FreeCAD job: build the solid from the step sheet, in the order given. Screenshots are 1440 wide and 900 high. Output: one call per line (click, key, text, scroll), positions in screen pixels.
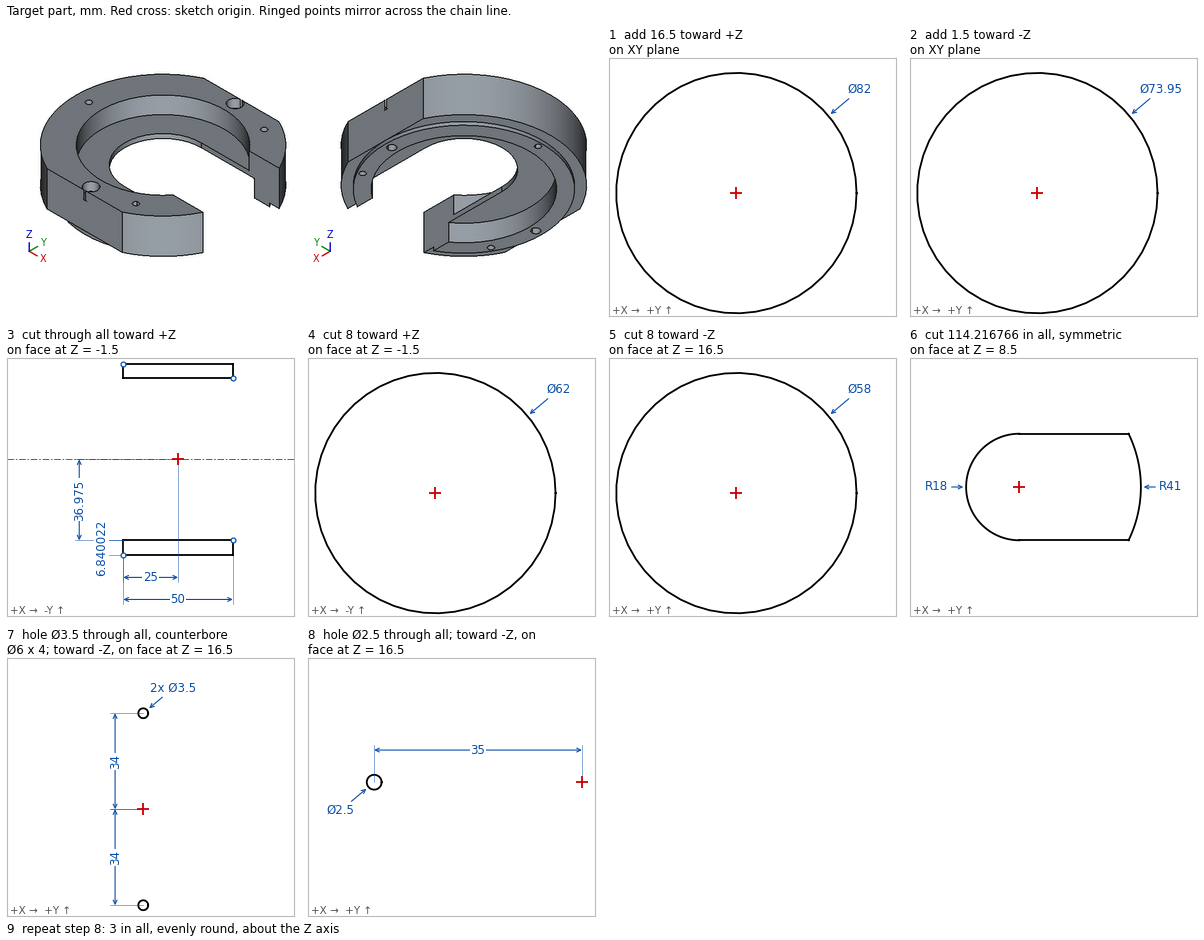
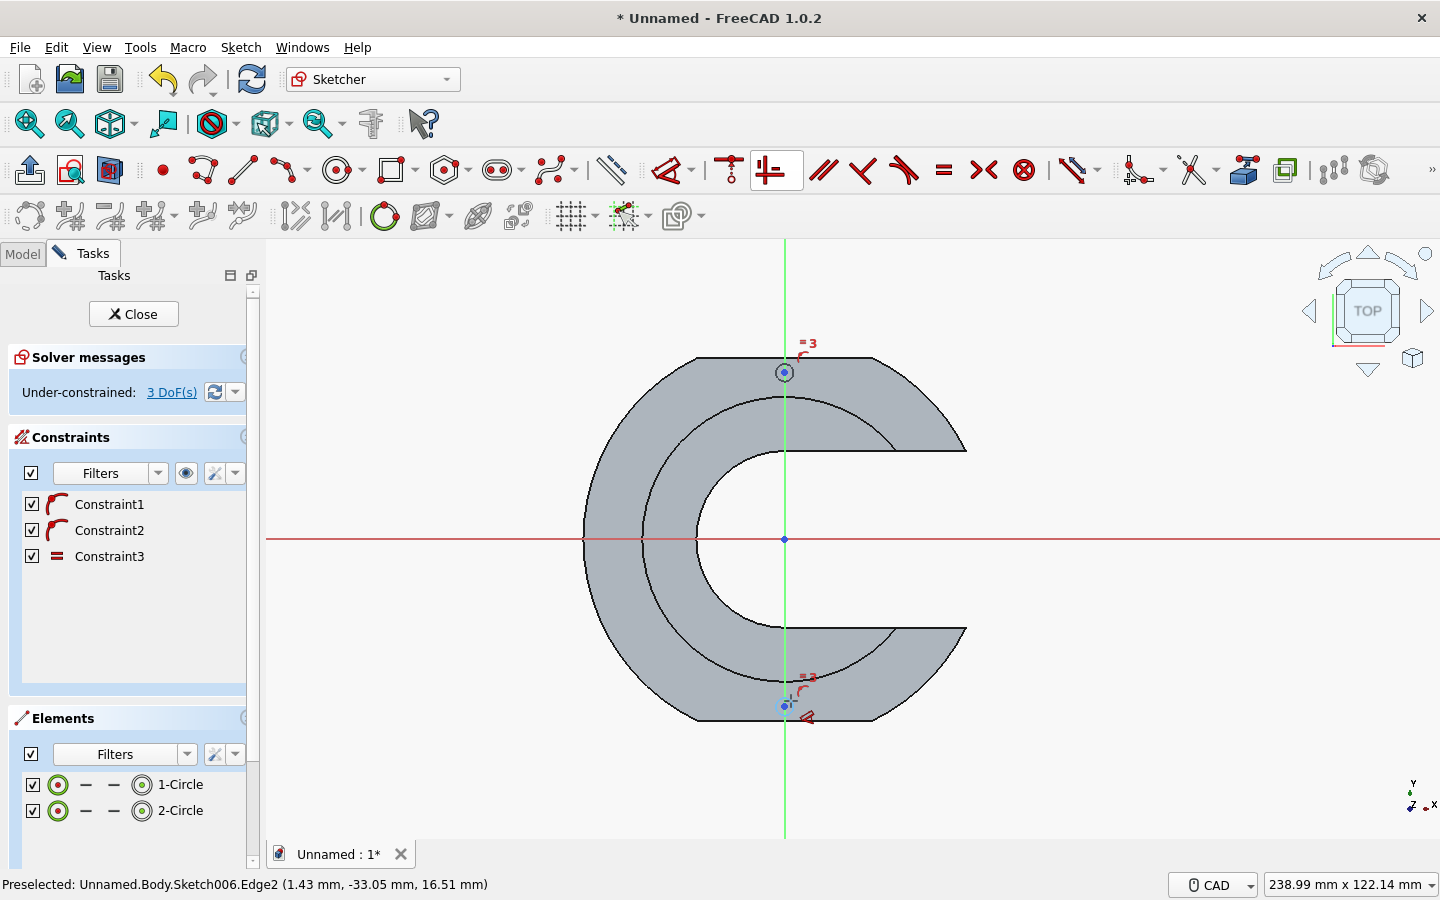
scroll(791, 367, up, 5)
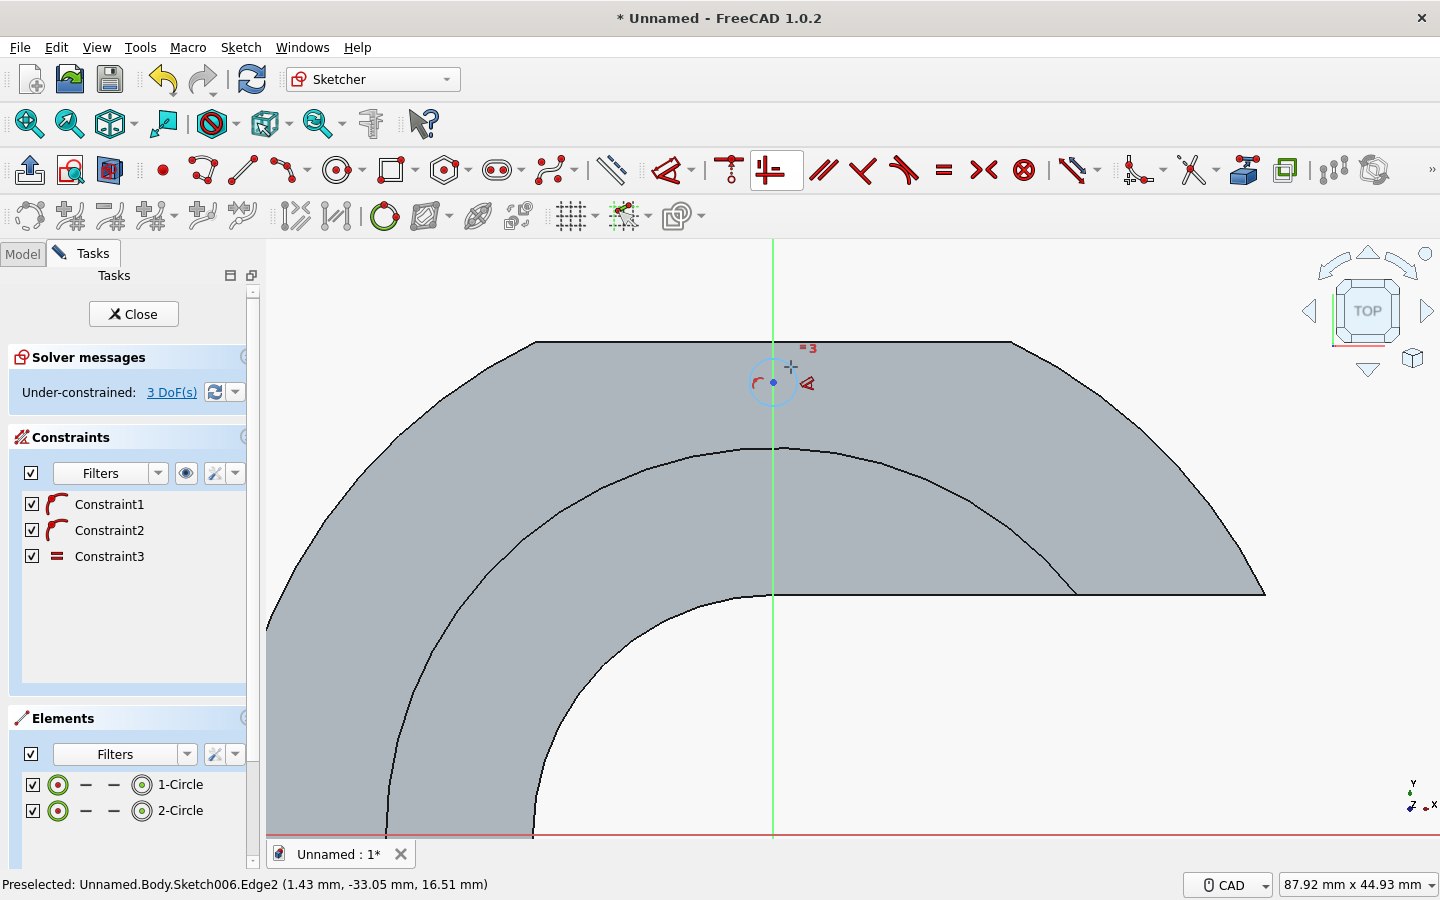
click(790, 366)
click(813, 344)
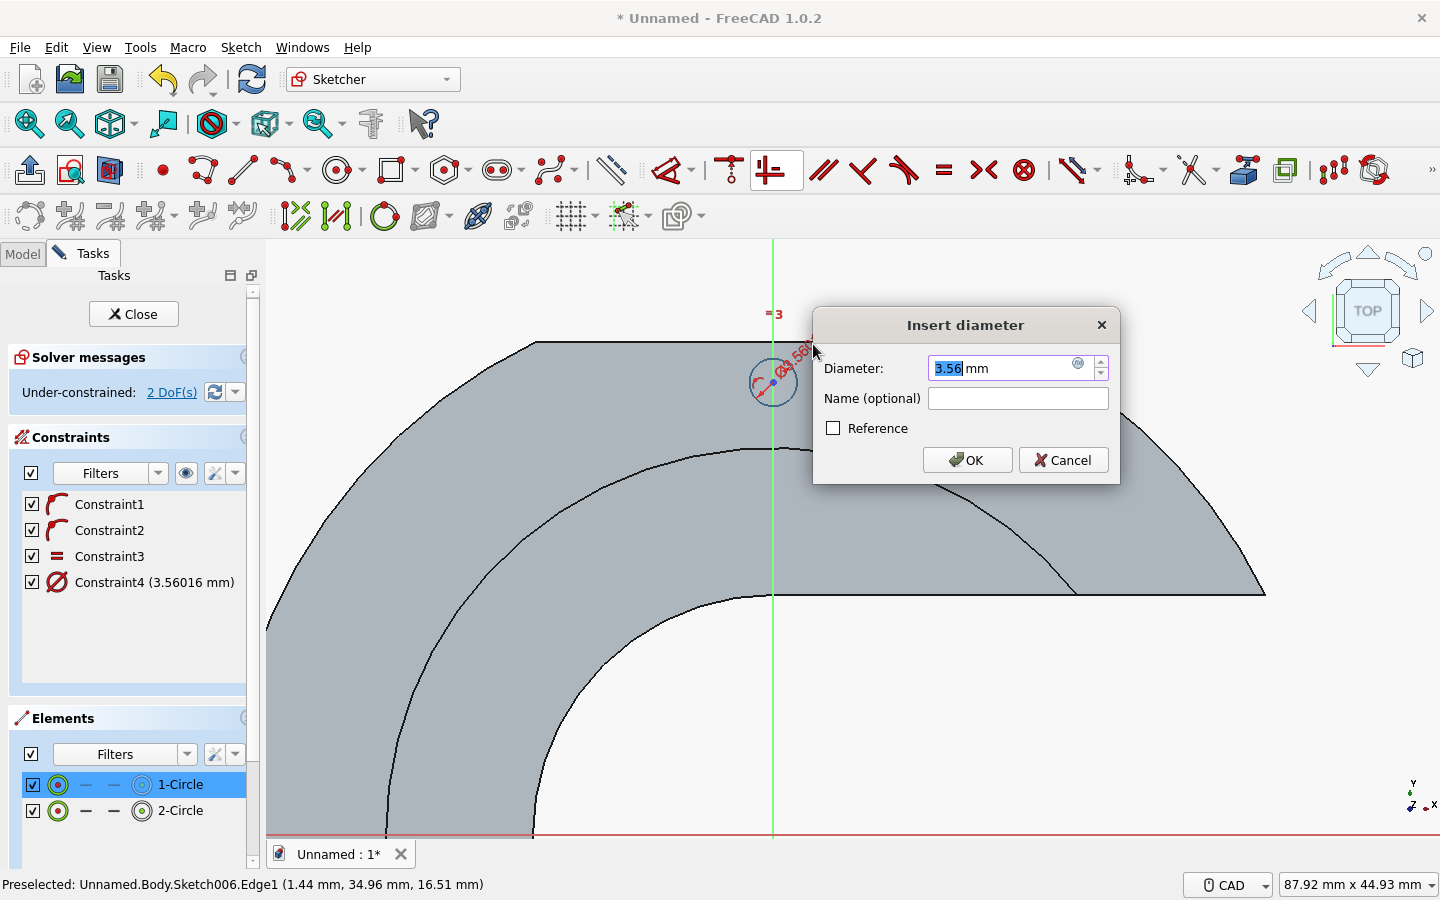
text(3.5)
key(Return)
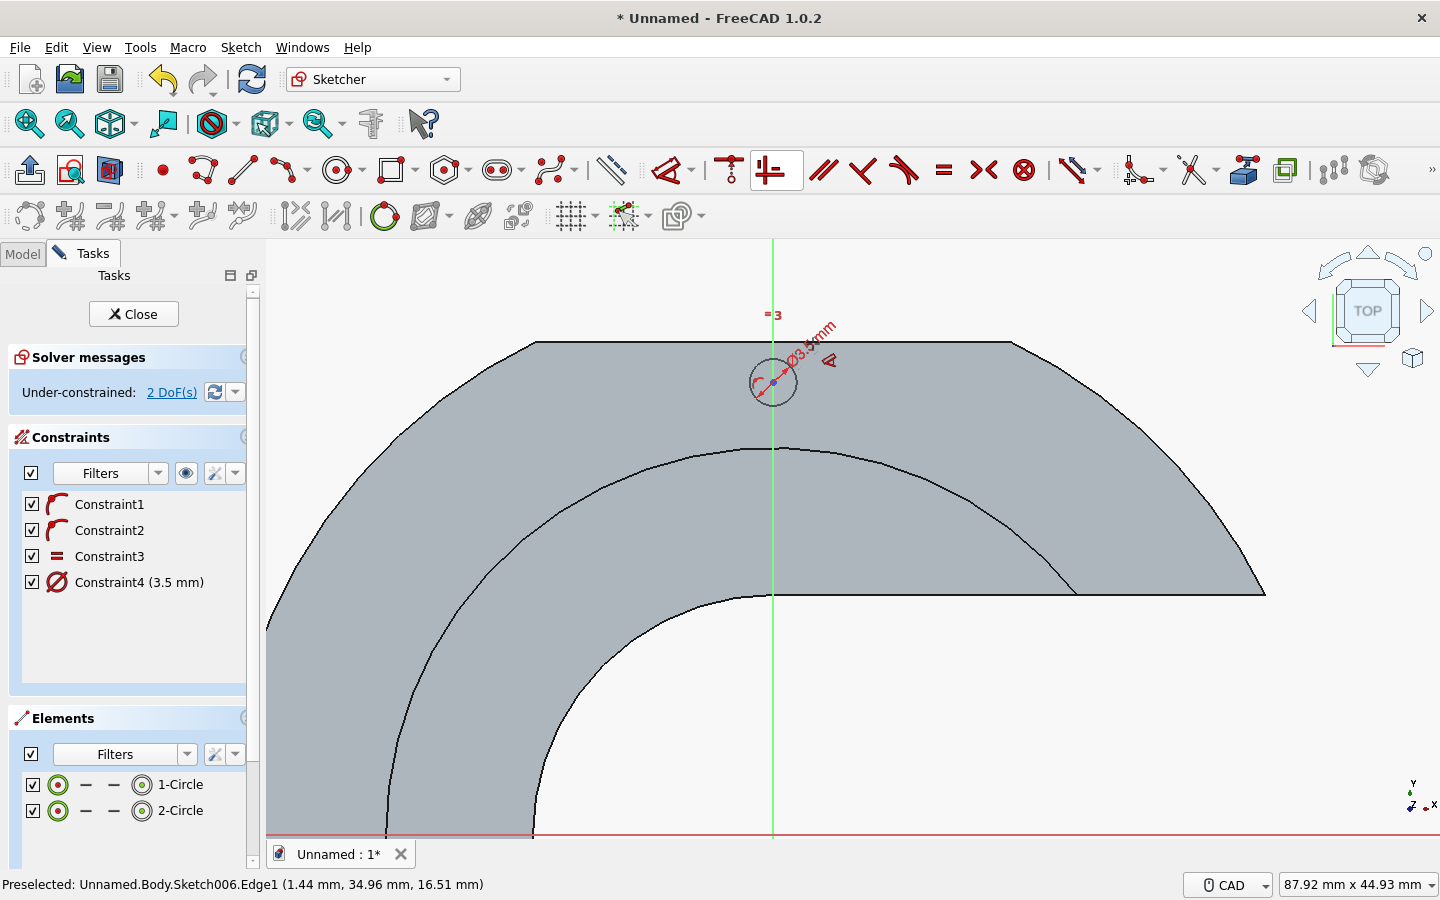
click(773, 382)
click(807, 597)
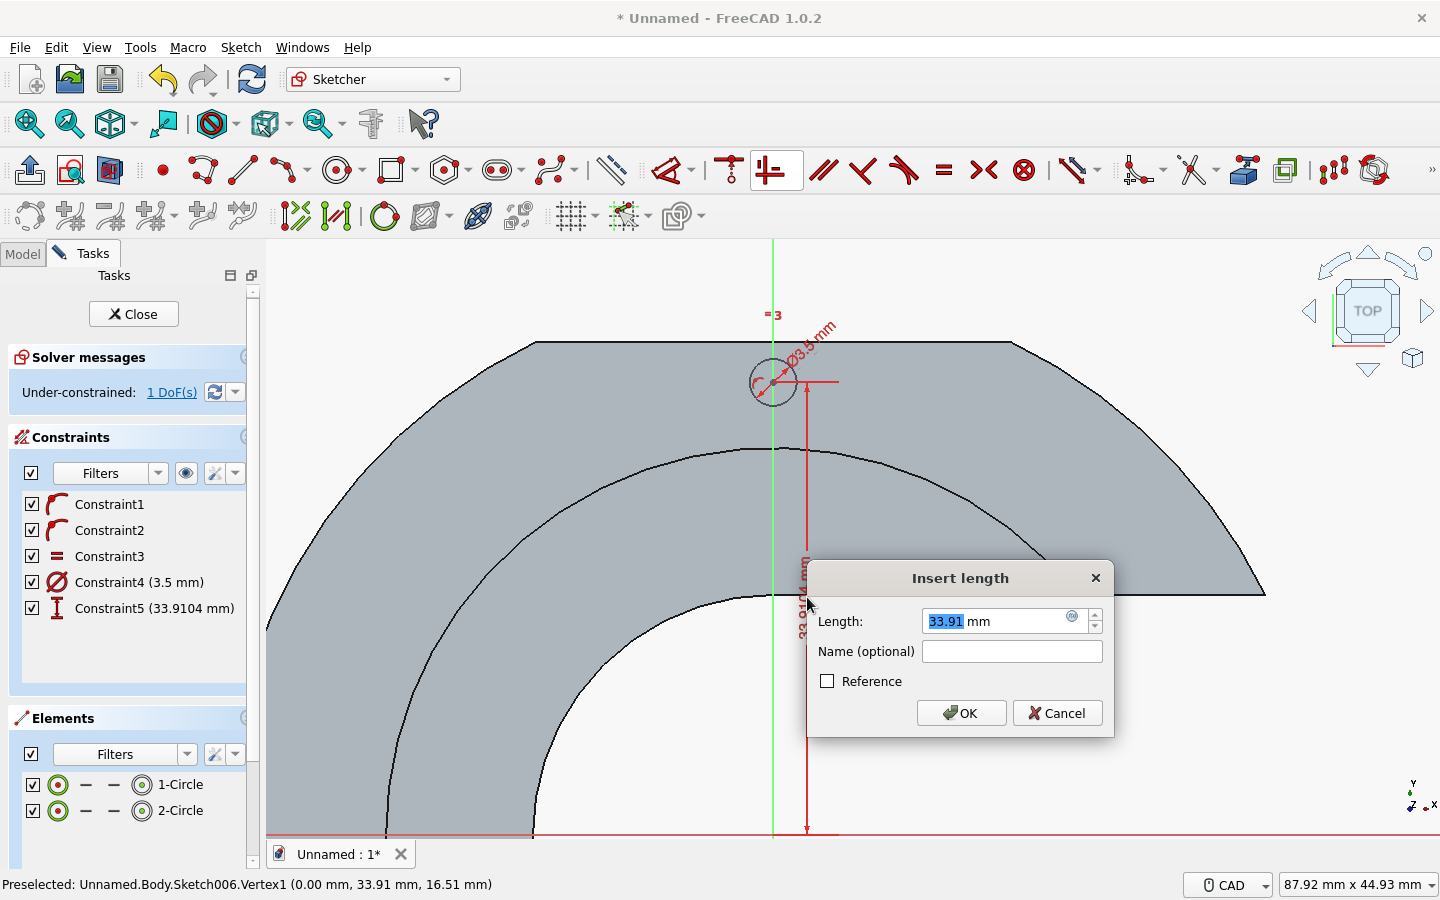
text(34)
key(Return)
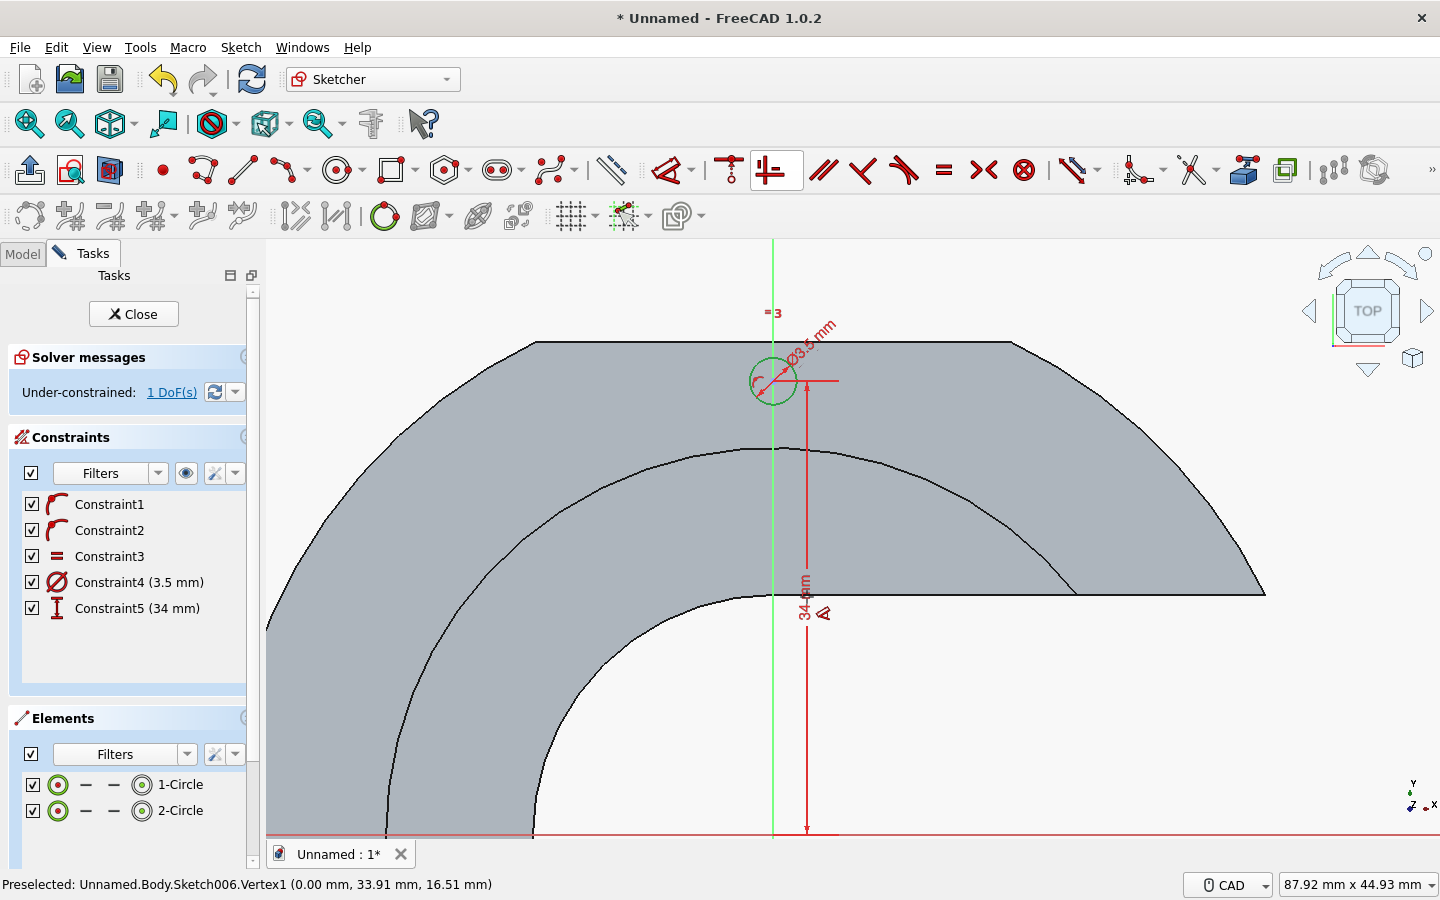
scroll(791, 367, down, 5)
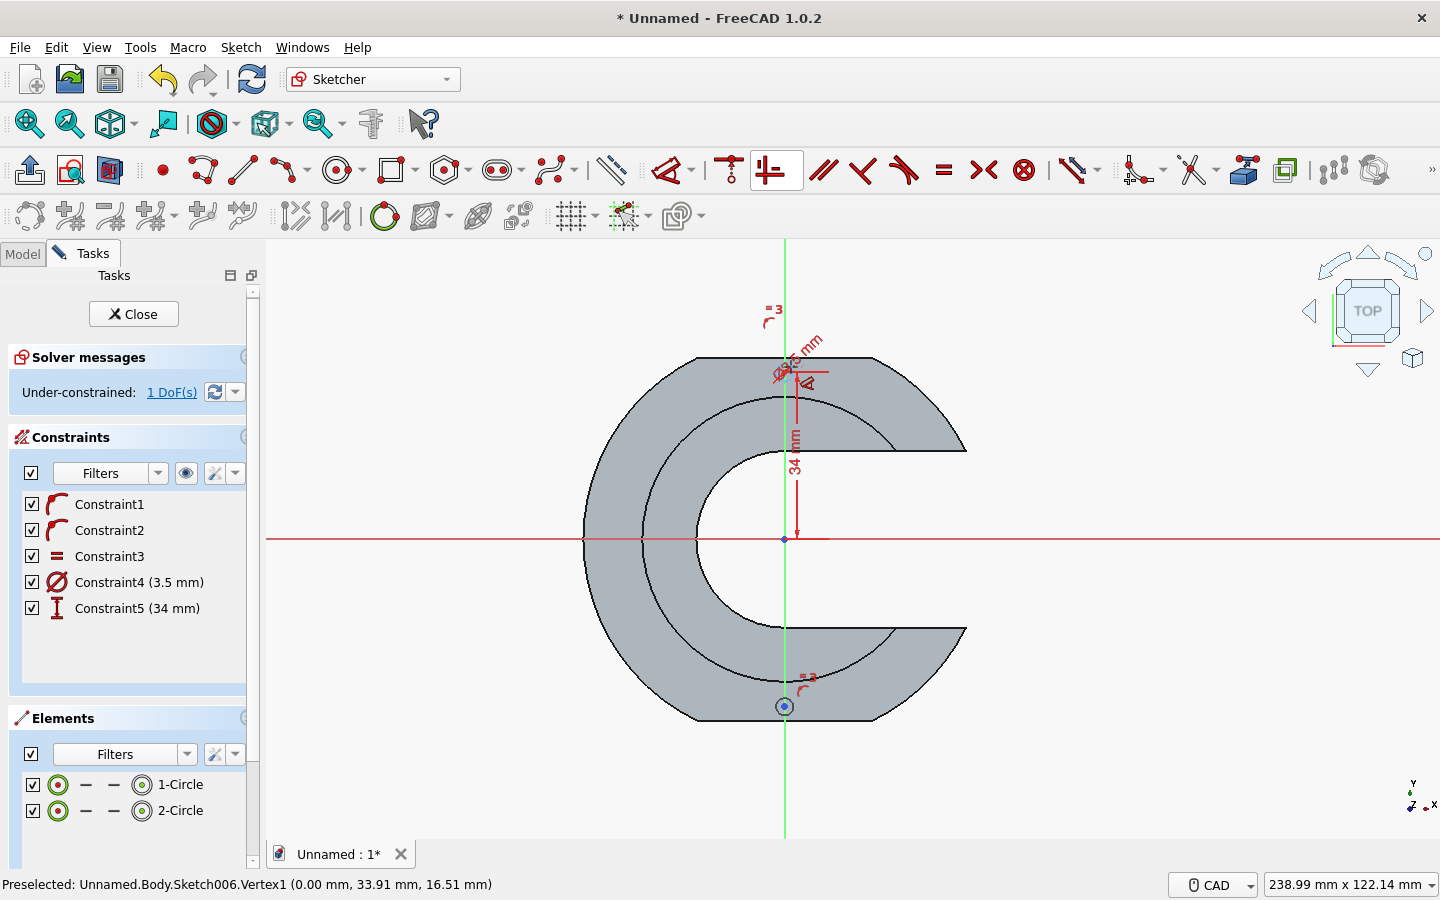
click(785, 707)
click(819, 623)